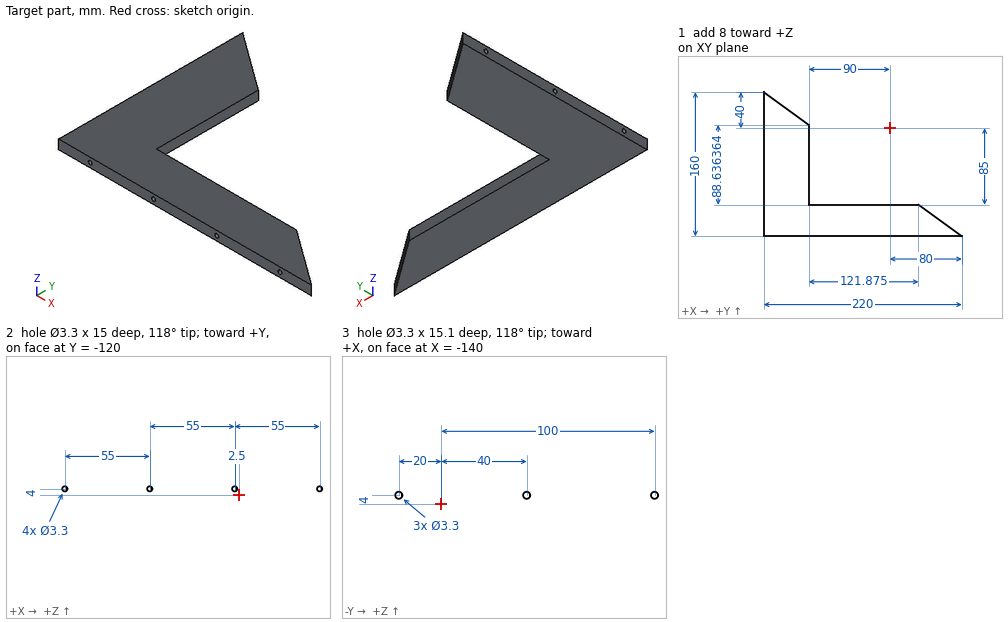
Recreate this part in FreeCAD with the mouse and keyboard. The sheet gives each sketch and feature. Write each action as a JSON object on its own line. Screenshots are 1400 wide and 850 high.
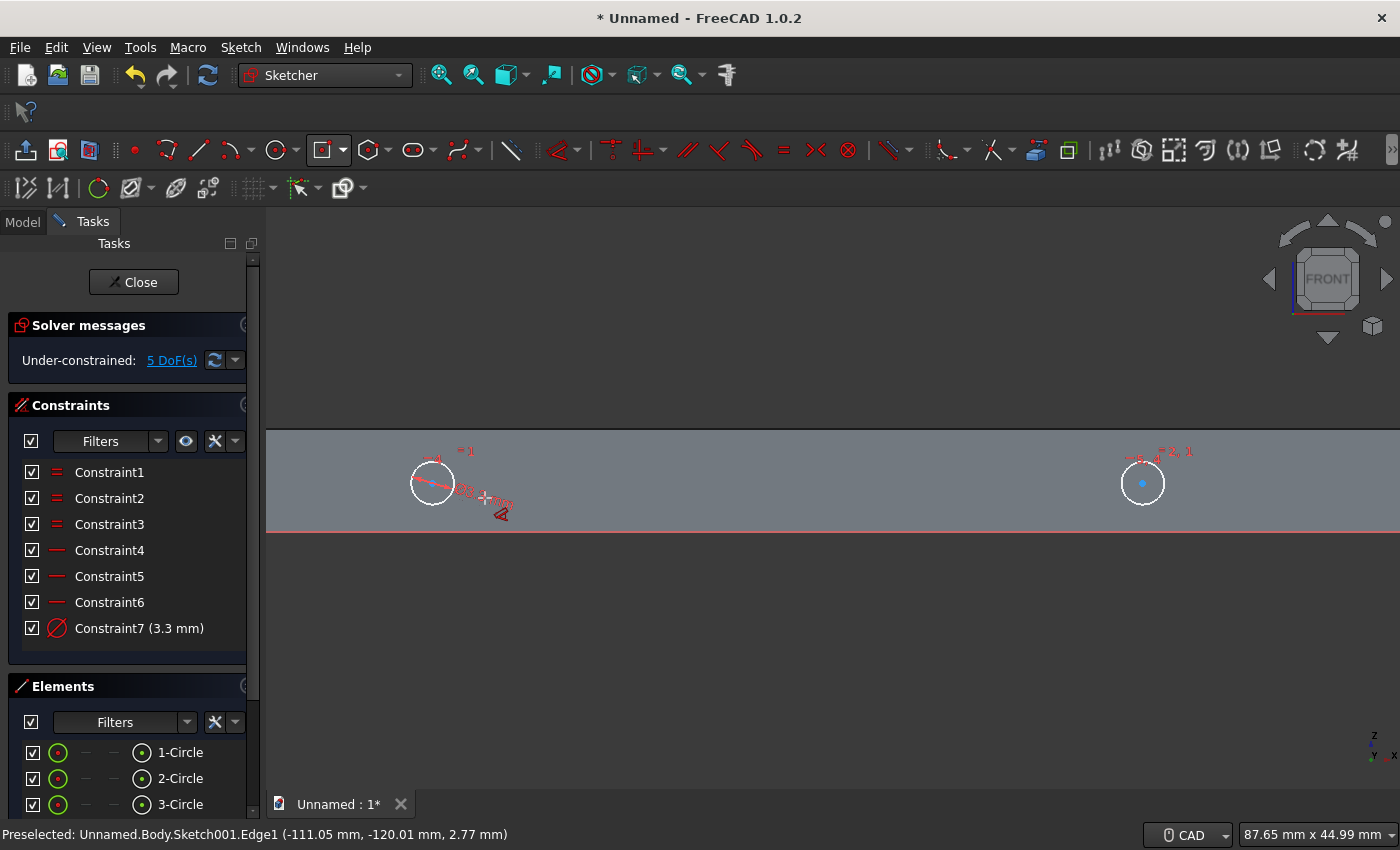
{"action": "left_click", "coordinate": [433, 483]}
{"action": "left_click", "coordinate": [399, 508]}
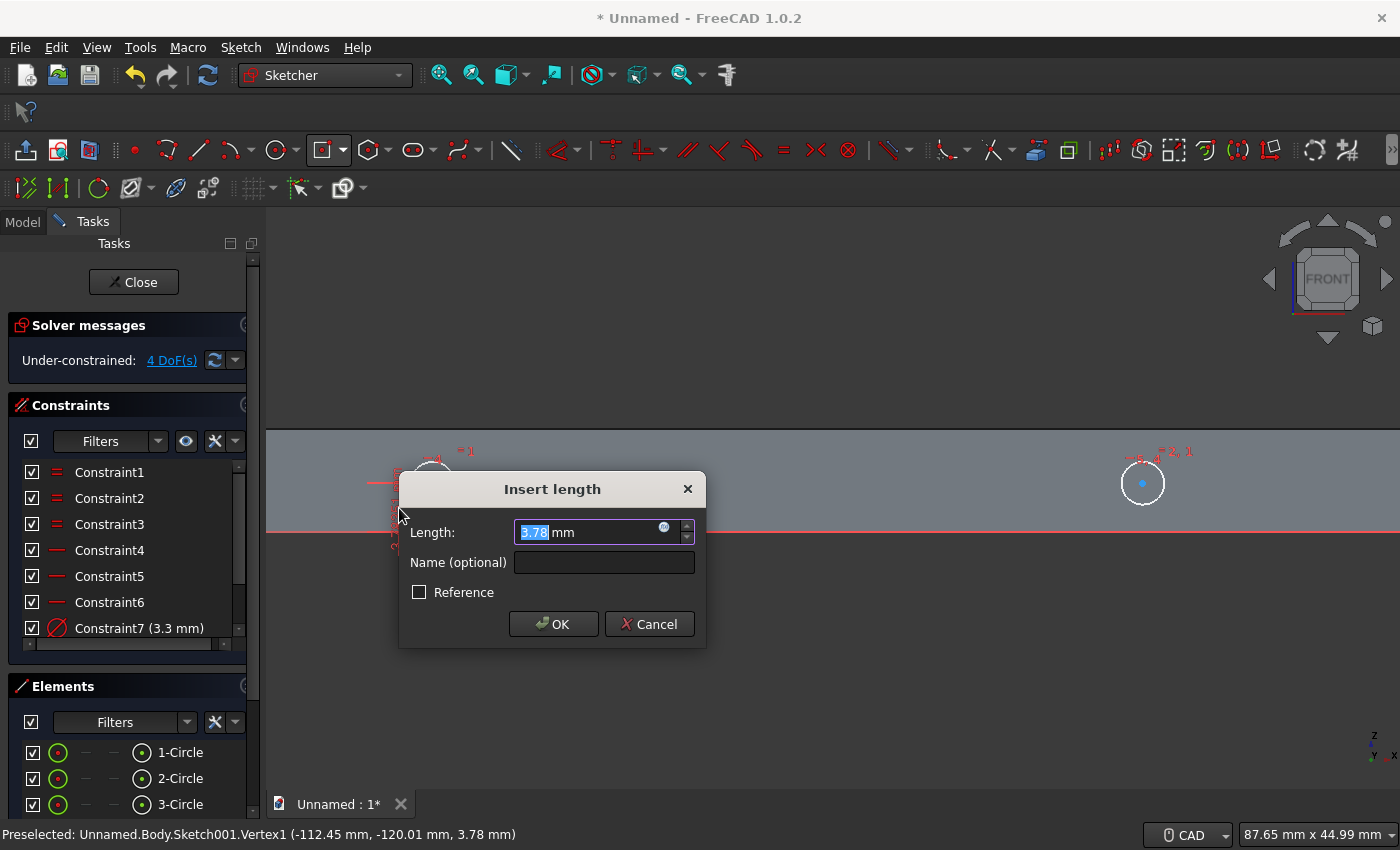
{"action": "type", "text": "4"}
{"action": "key", "text": "Return"}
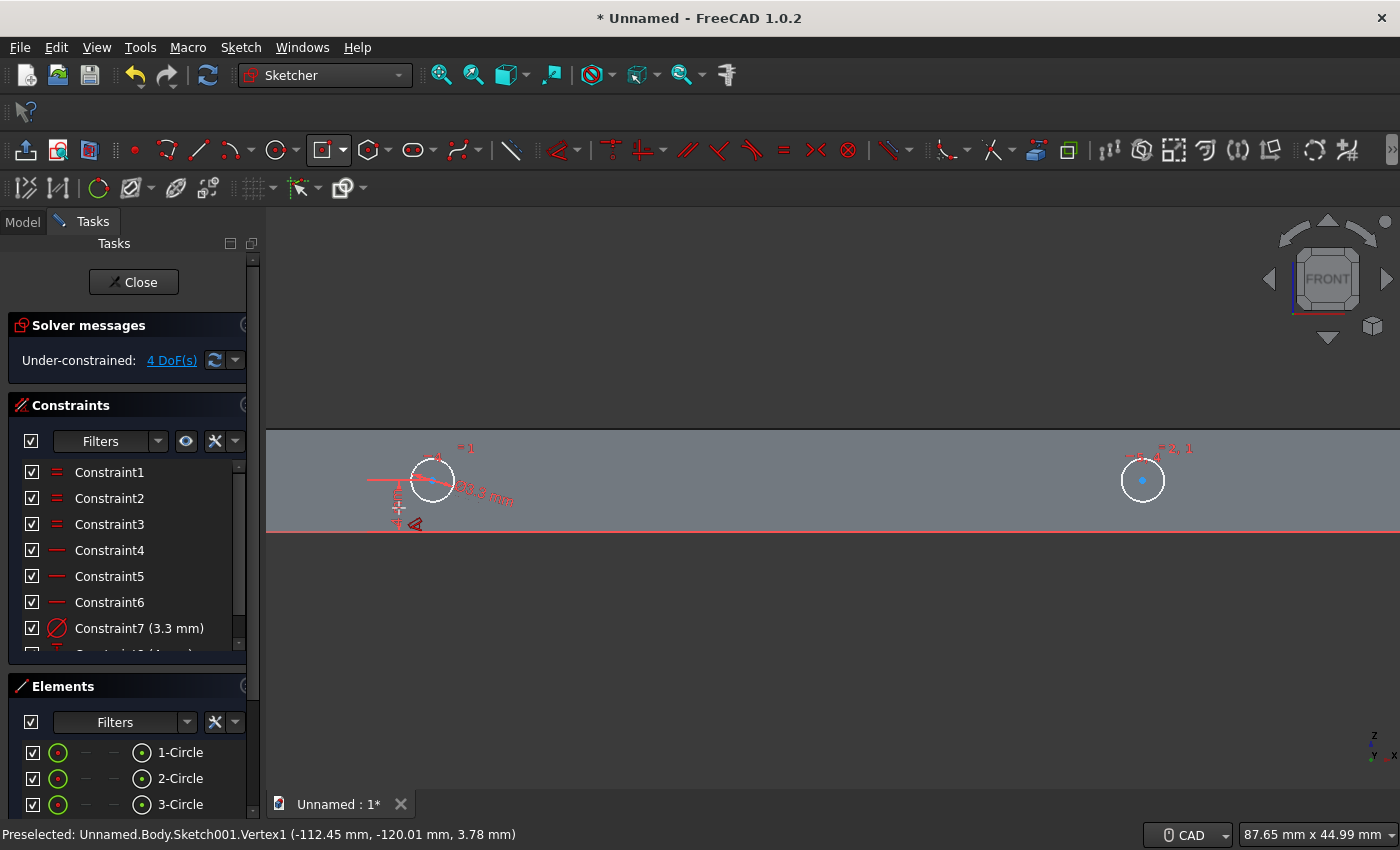
{"action": "scroll", "coordinate": [448, 499], "scroll_direction": "down", "scroll_amount": 6}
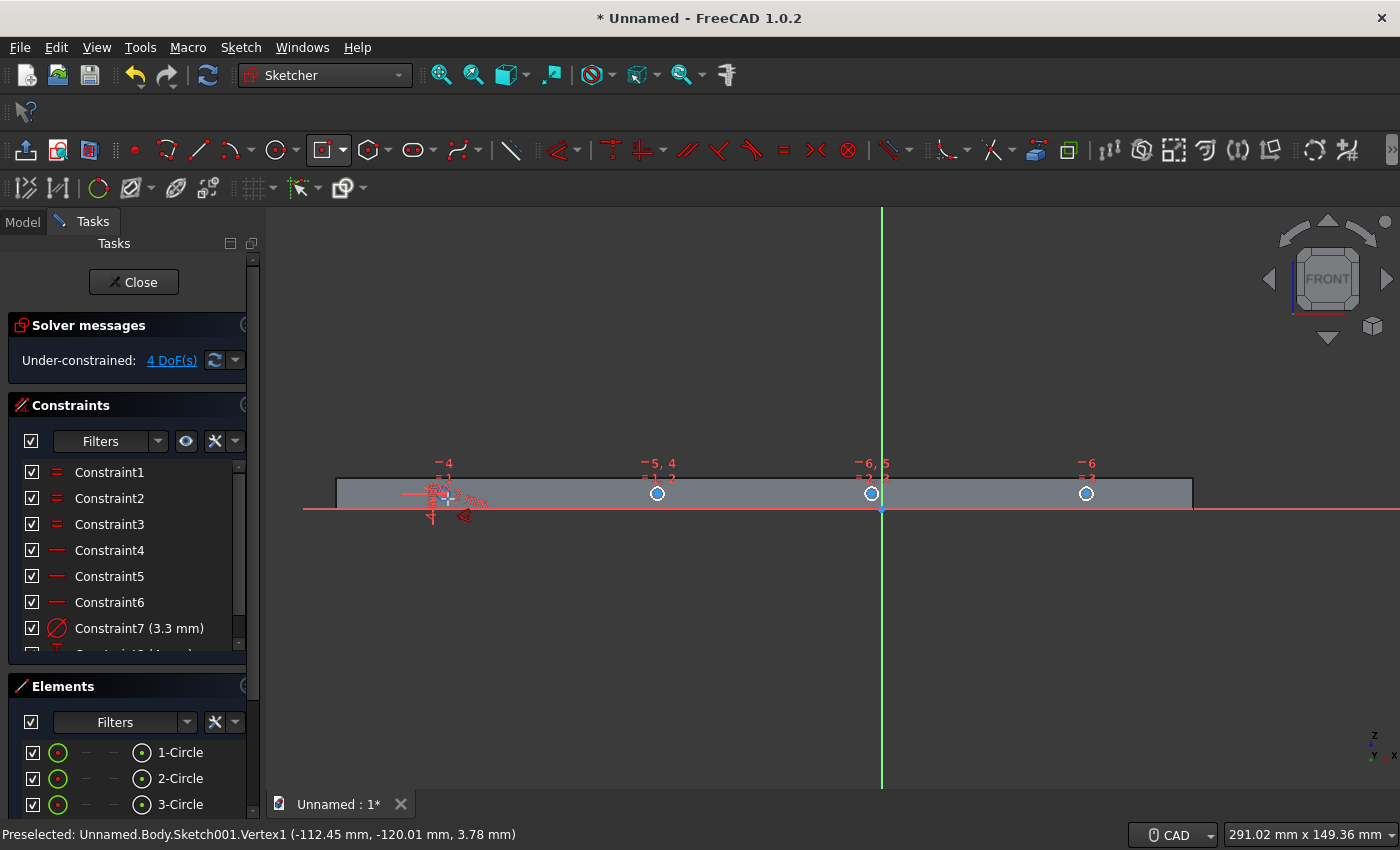
{"action": "scroll", "coordinate": [872, 494], "scroll_direction": "up", "scroll_amount": 8}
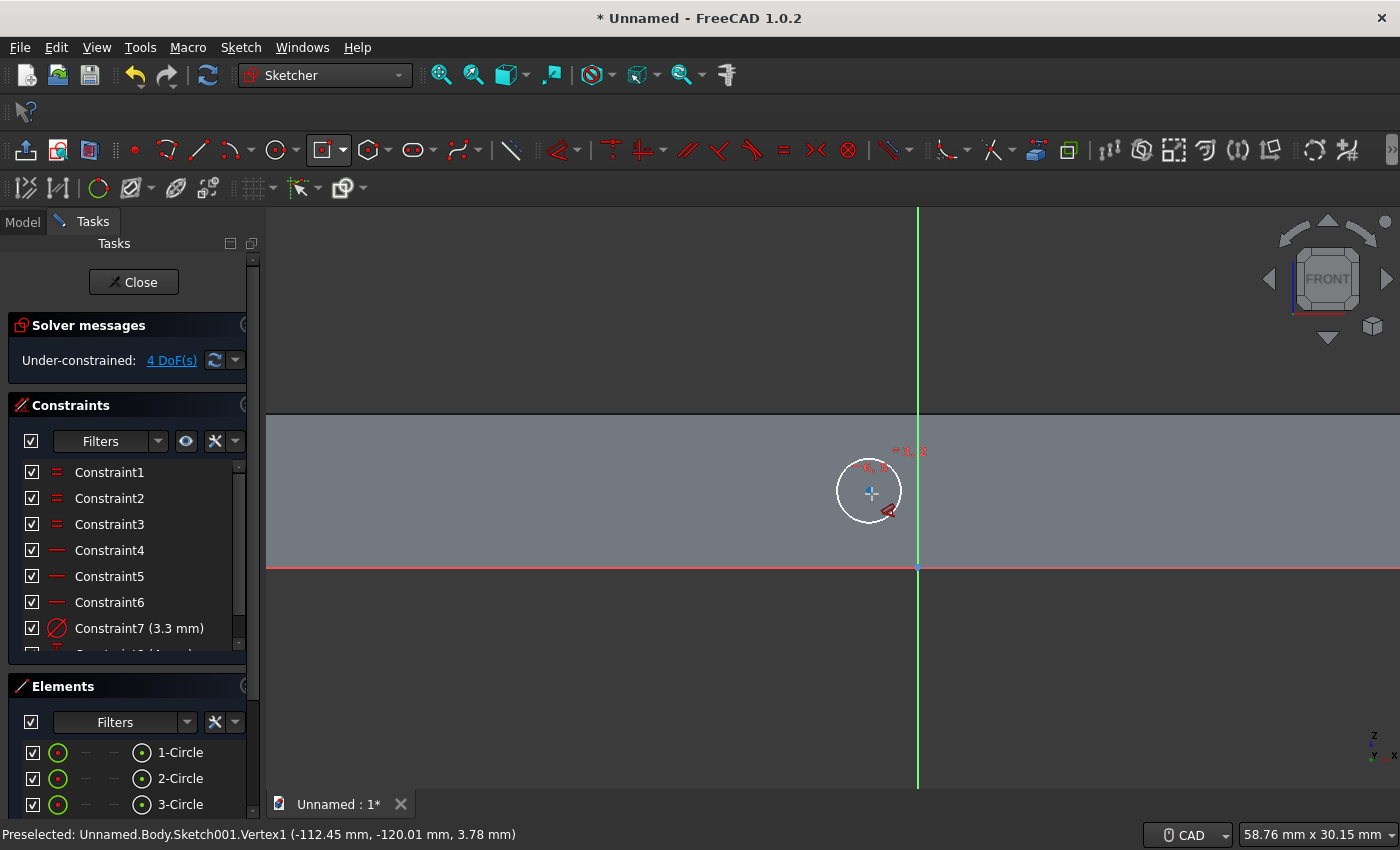
{"action": "left_click", "coordinate": [869, 491]}
{"action": "left_click", "coordinate": [893, 602]}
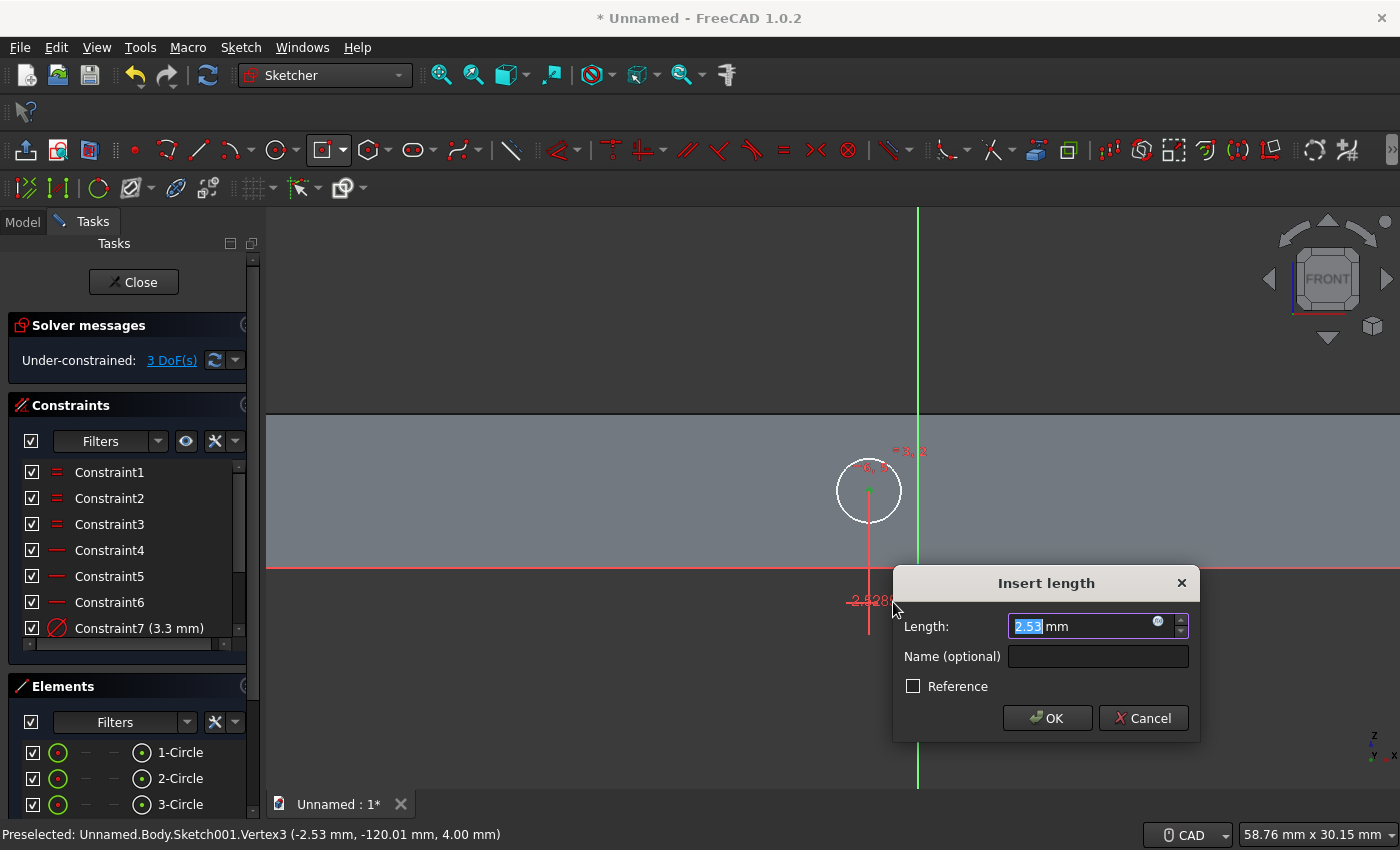
{"action": "type", "text": "2.5"}
{"action": "key", "text": "Return"}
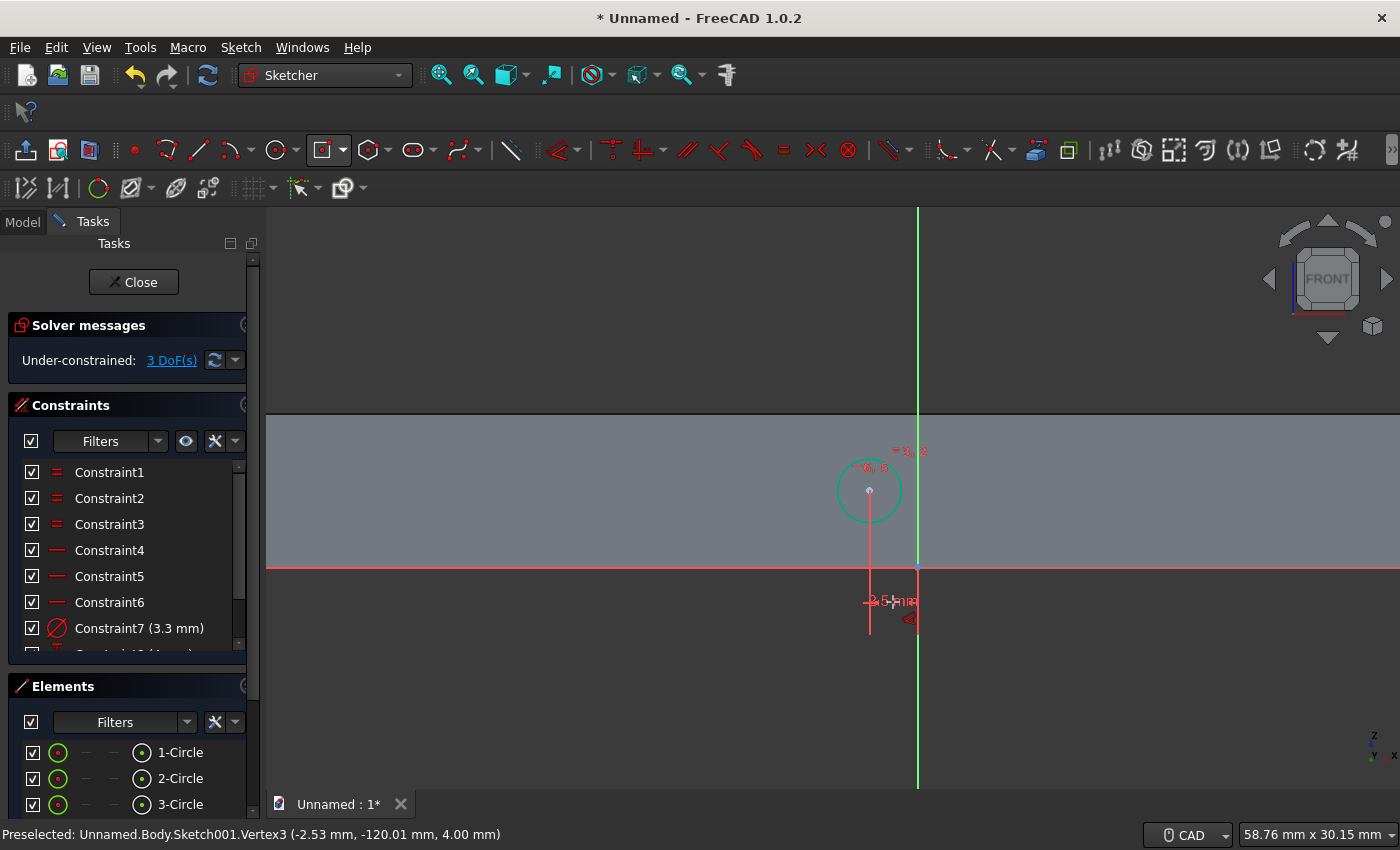
{"action": "scroll", "coordinate": [872, 494], "scroll_direction": "down", "scroll_amount": 8}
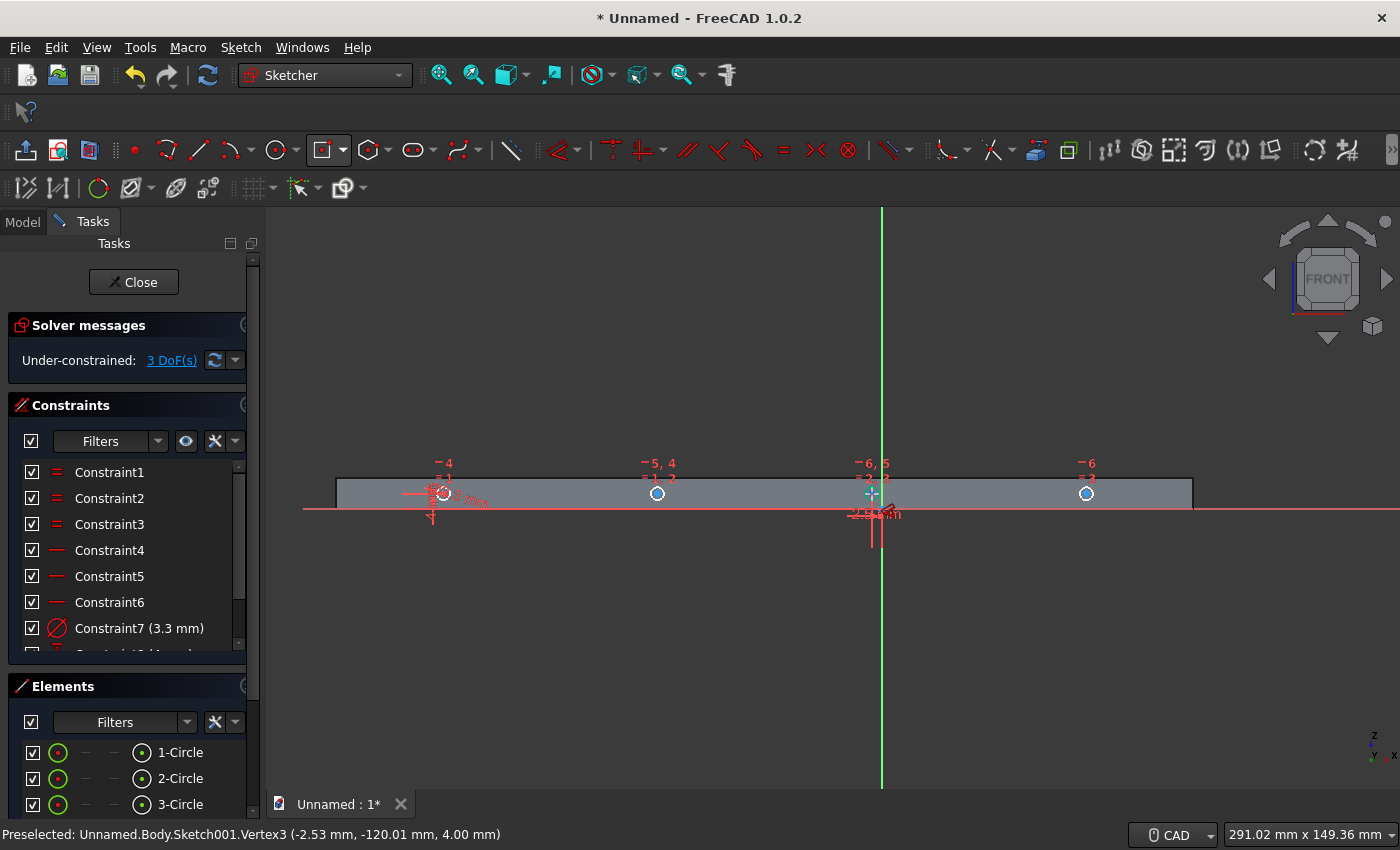
{"action": "left_click", "coordinate": [443, 494]}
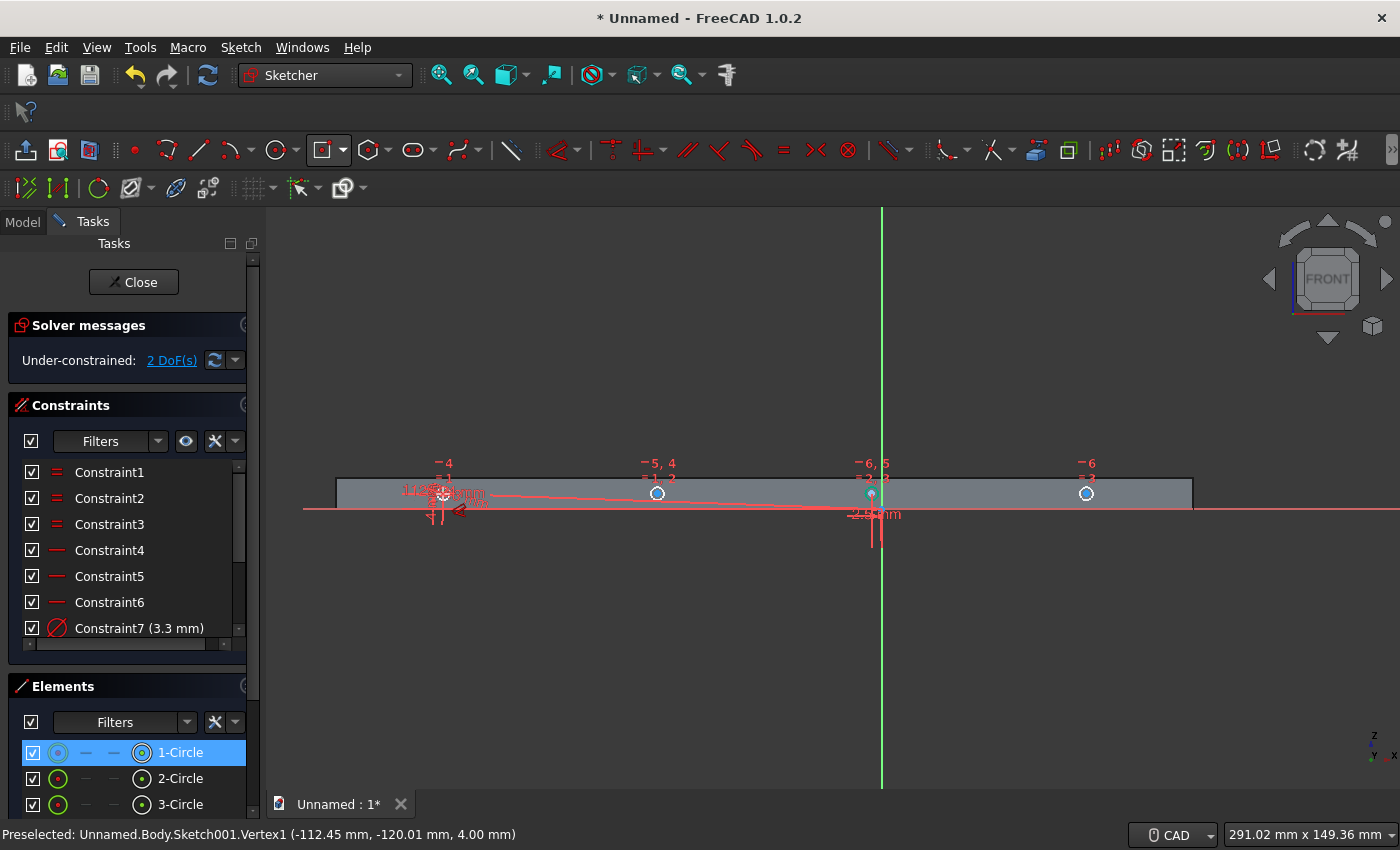
{"action": "left_click", "coordinate": [657, 494]}
{"action": "left_click", "coordinate": [550, 460]}